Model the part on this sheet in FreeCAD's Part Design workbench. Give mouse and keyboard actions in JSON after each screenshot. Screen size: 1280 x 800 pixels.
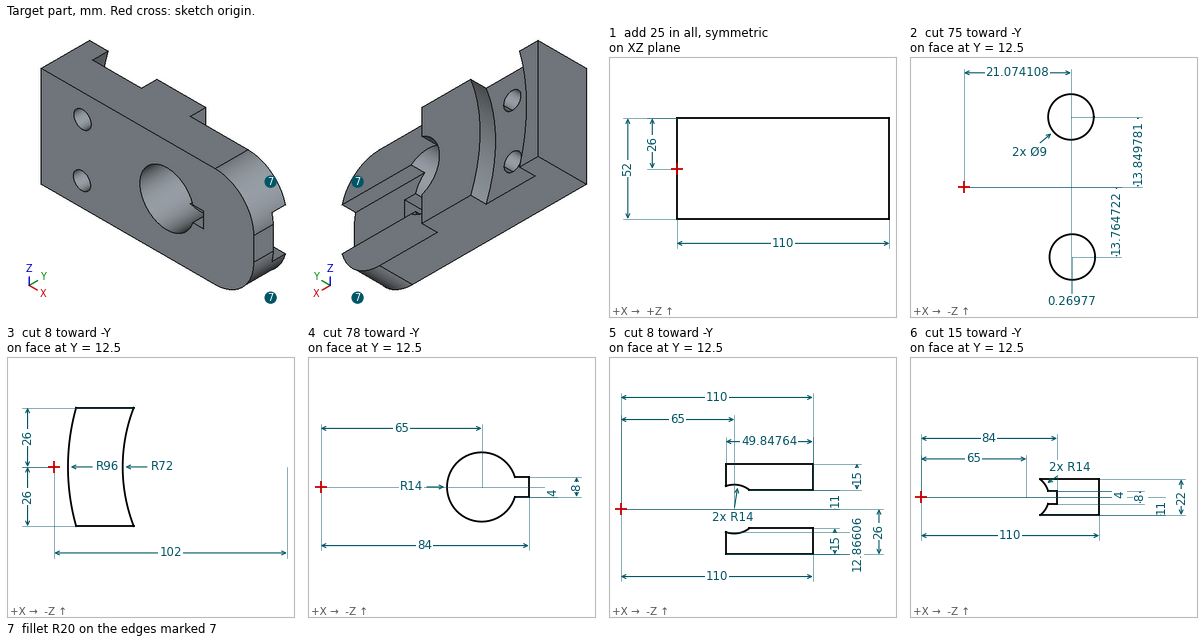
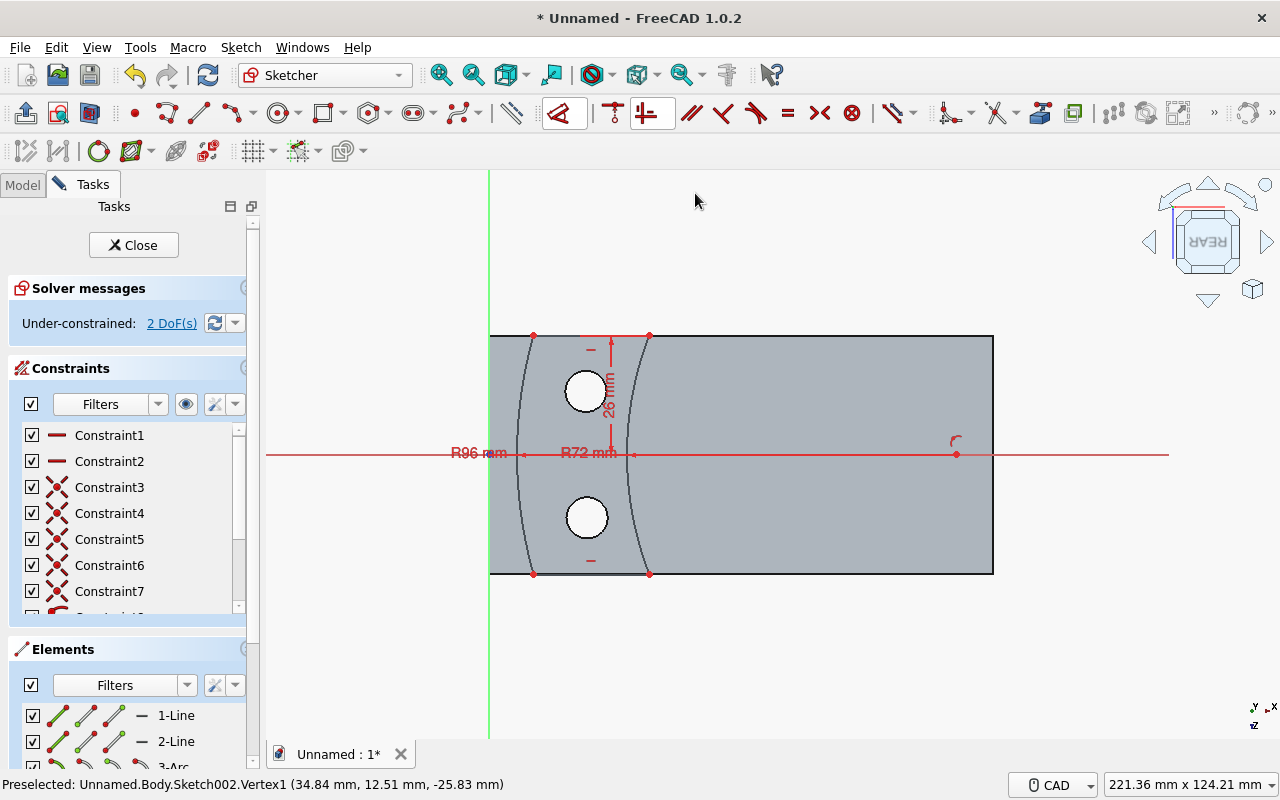
{"action": "left_click", "coordinate": [534, 575]}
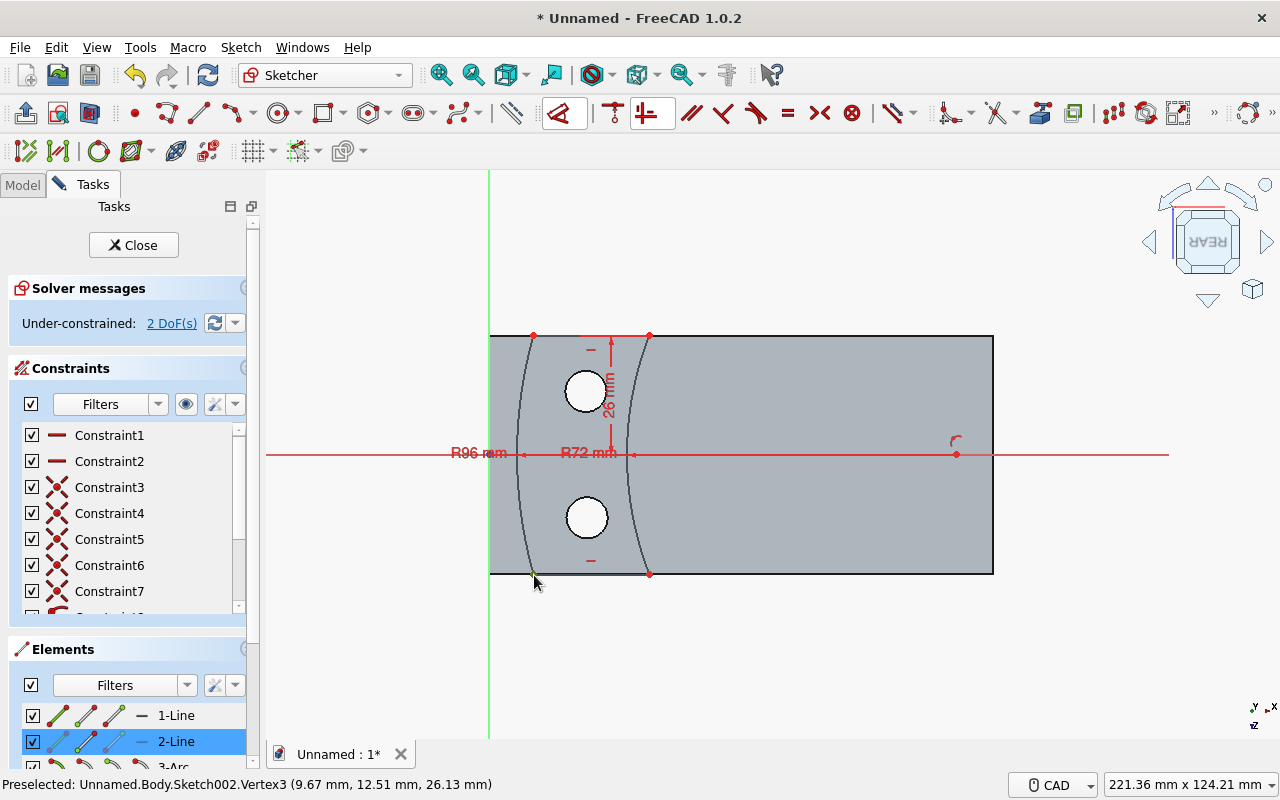
{"action": "key", "text": "i"}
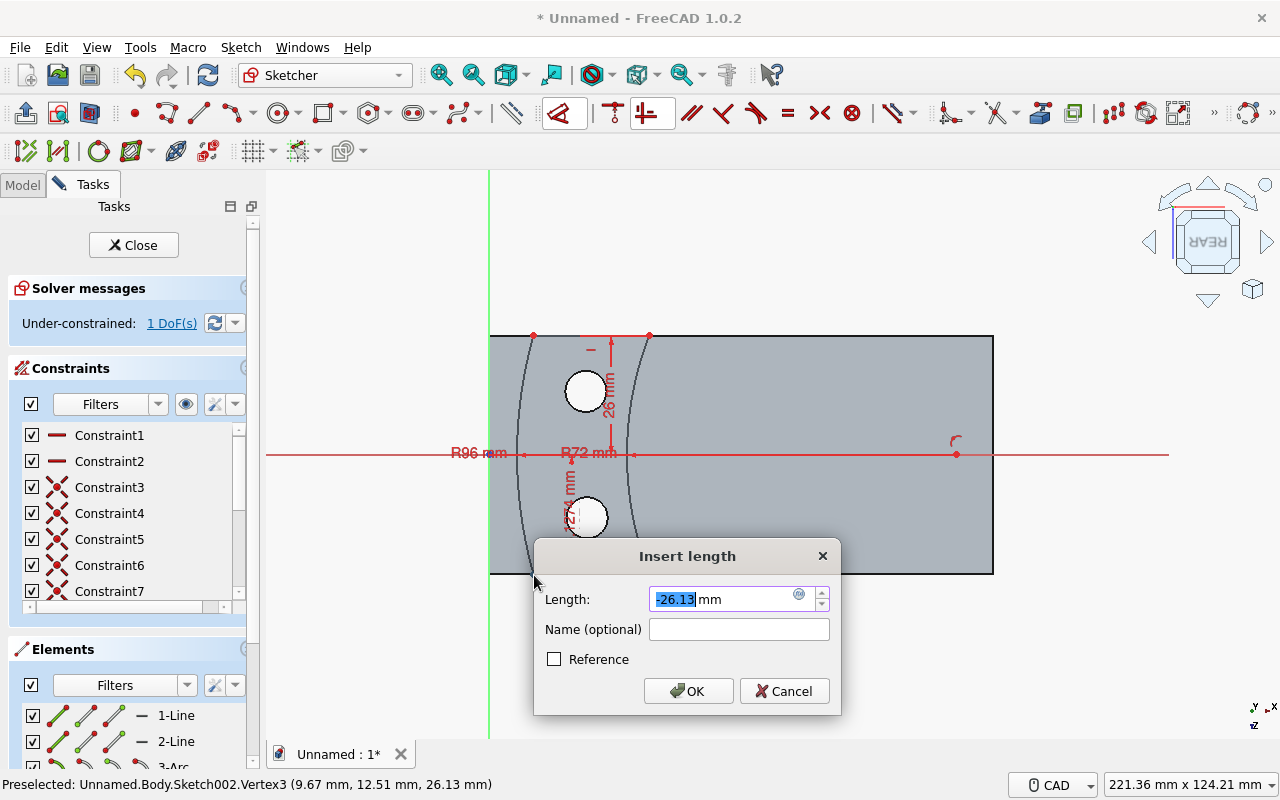
{"action": "type", "text": "-26"}
{"action": "key", "text": "Return"}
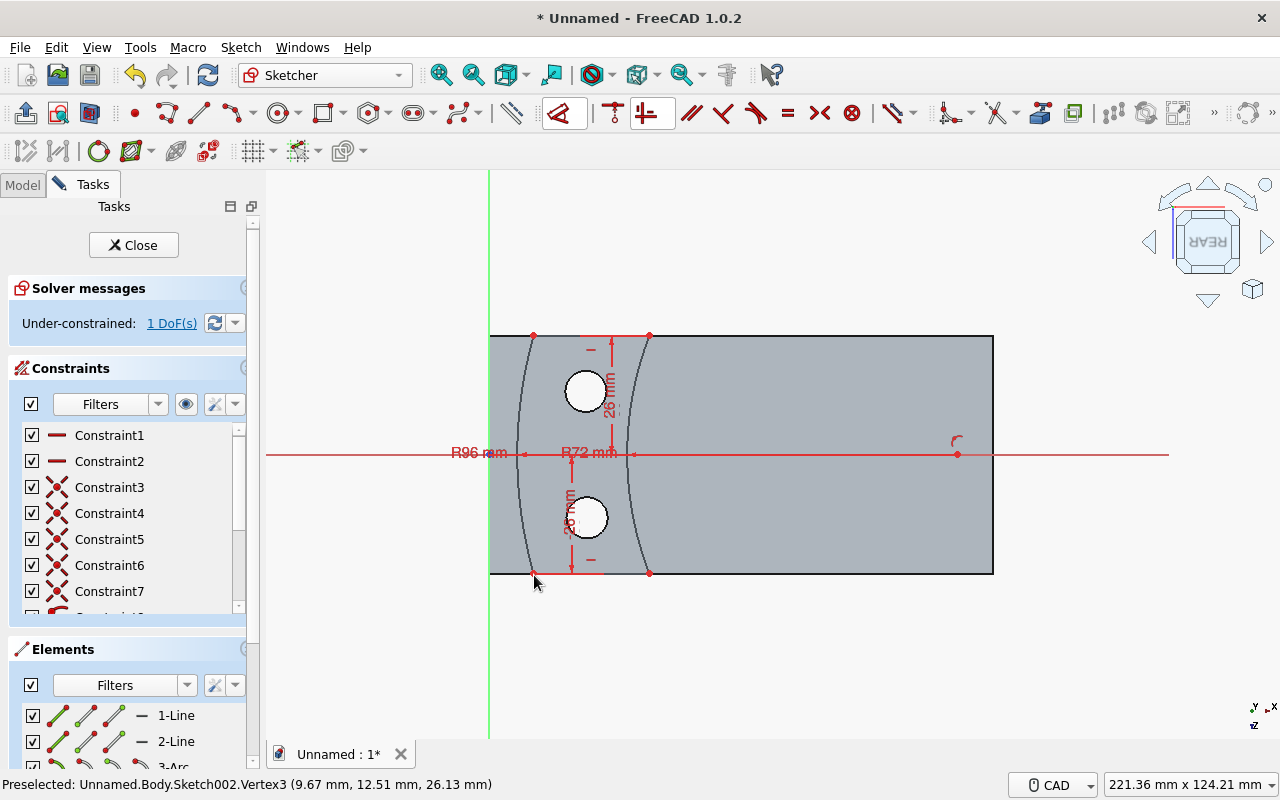
{"action": "left_click", "coordinate": [957, 455]}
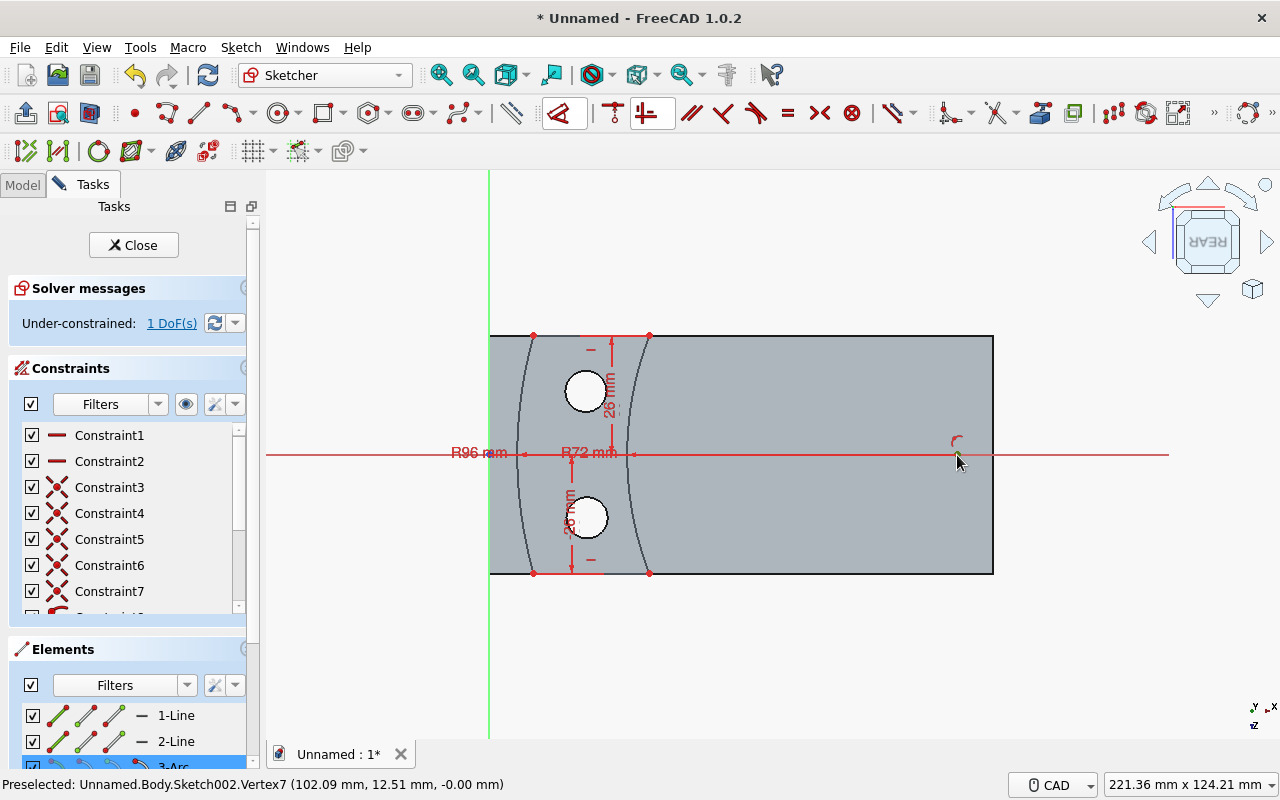
{"action": "left_click", "coordinate": [582, 114]}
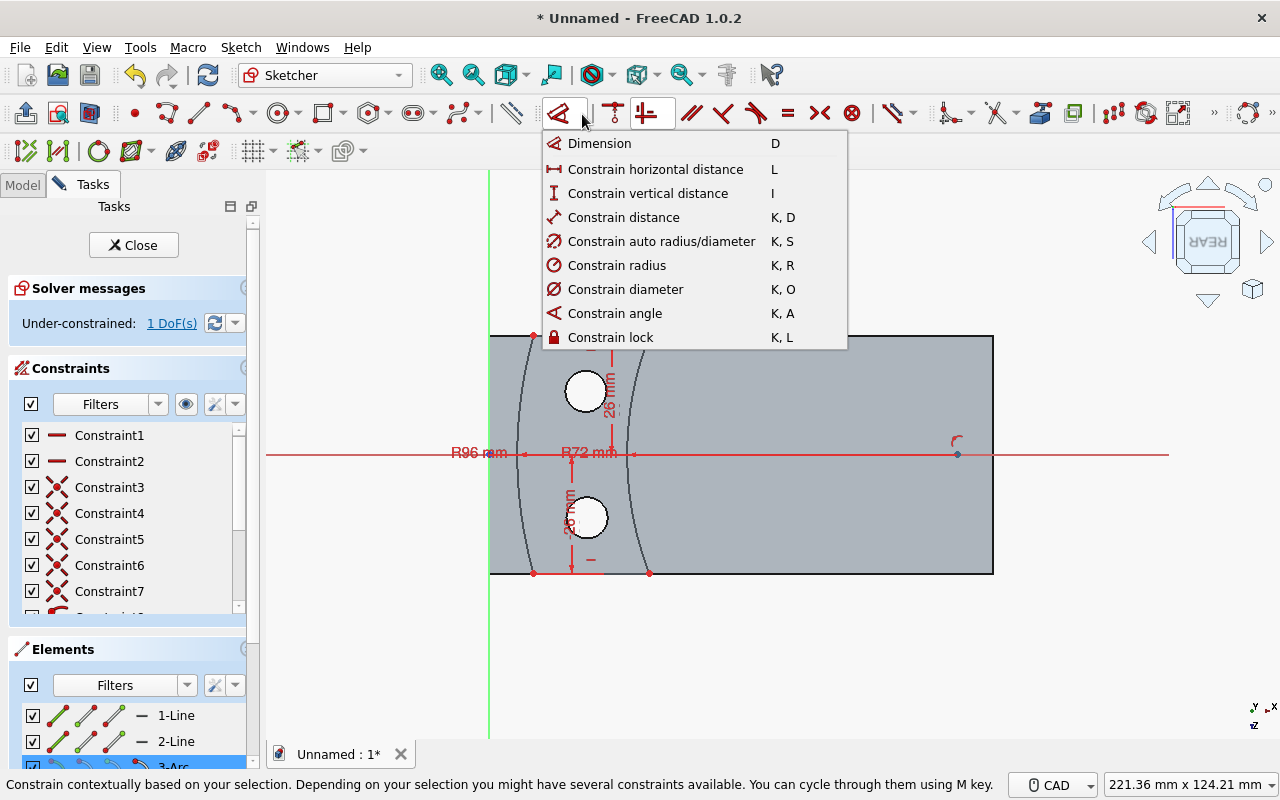
{"action": "left_click", "coordinate": [695, 169]}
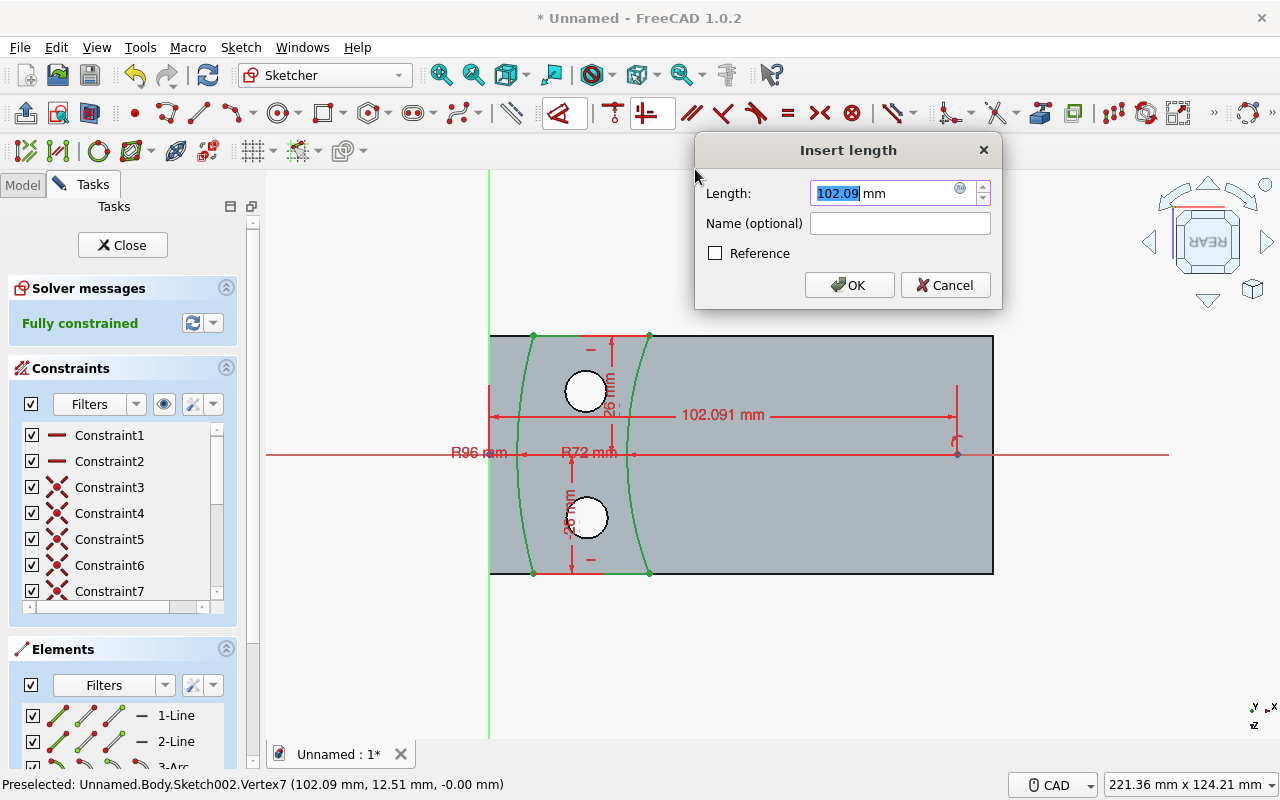
{"action": "type", "text": "102"}
{"action": "key", "text": "Return"}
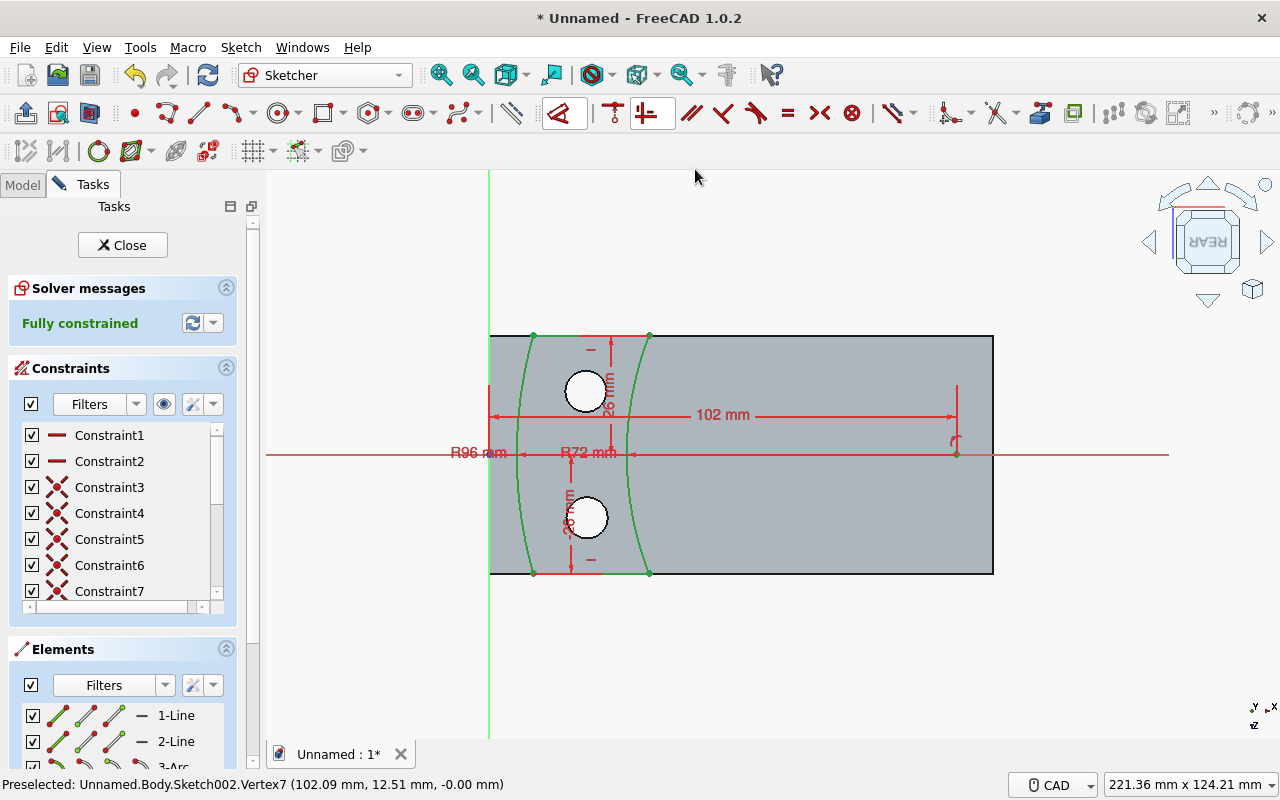
{"action": "left_click", "coordinate": [123, 245]}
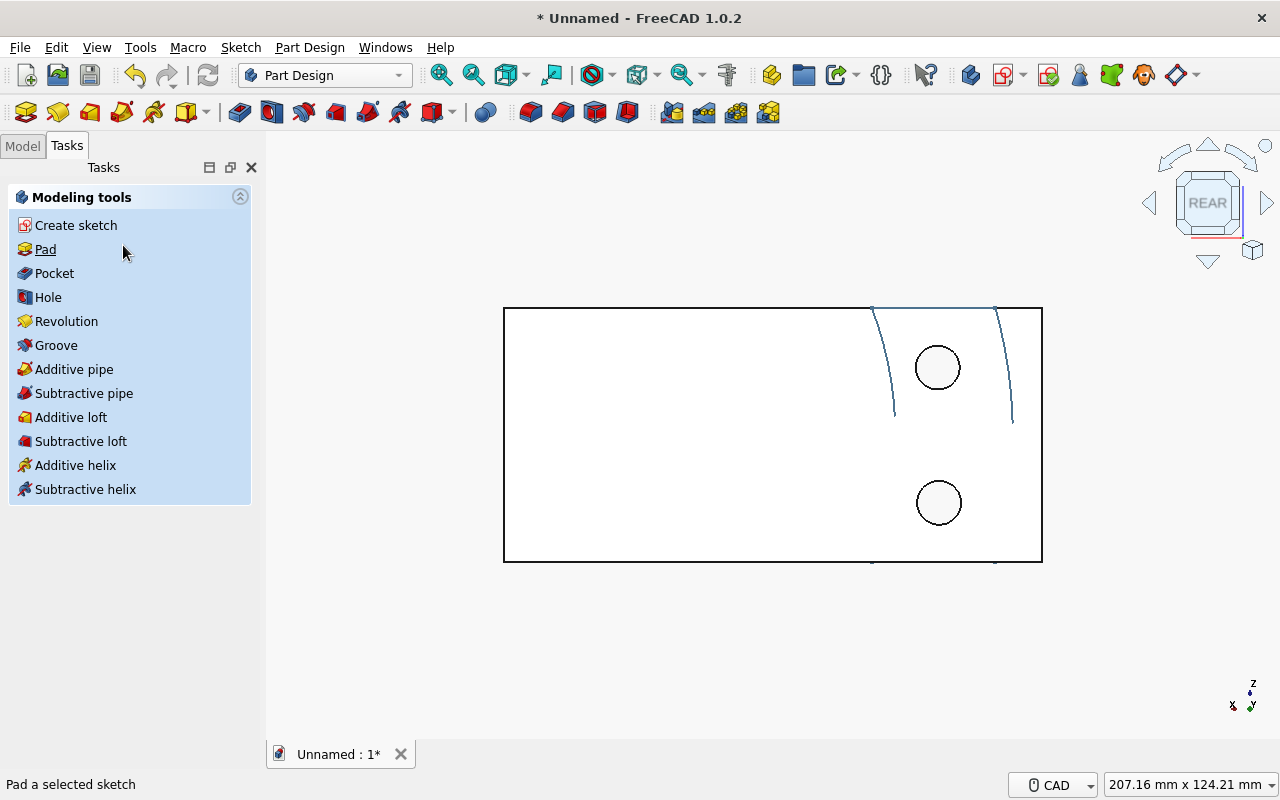
{"action": "left_click", "coordinate": [240, 112]}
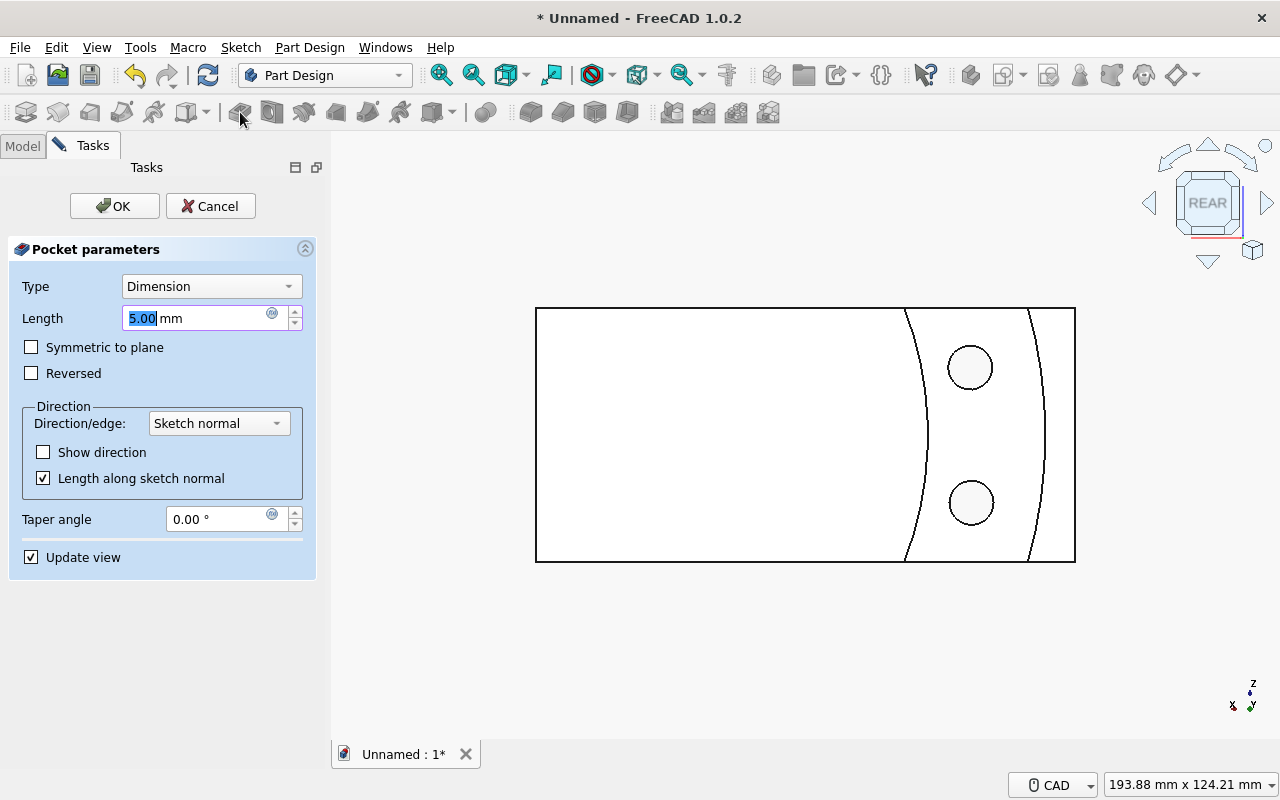
{"action": "type", "text": "8"}
{"action": "key", "text": "Tab"}